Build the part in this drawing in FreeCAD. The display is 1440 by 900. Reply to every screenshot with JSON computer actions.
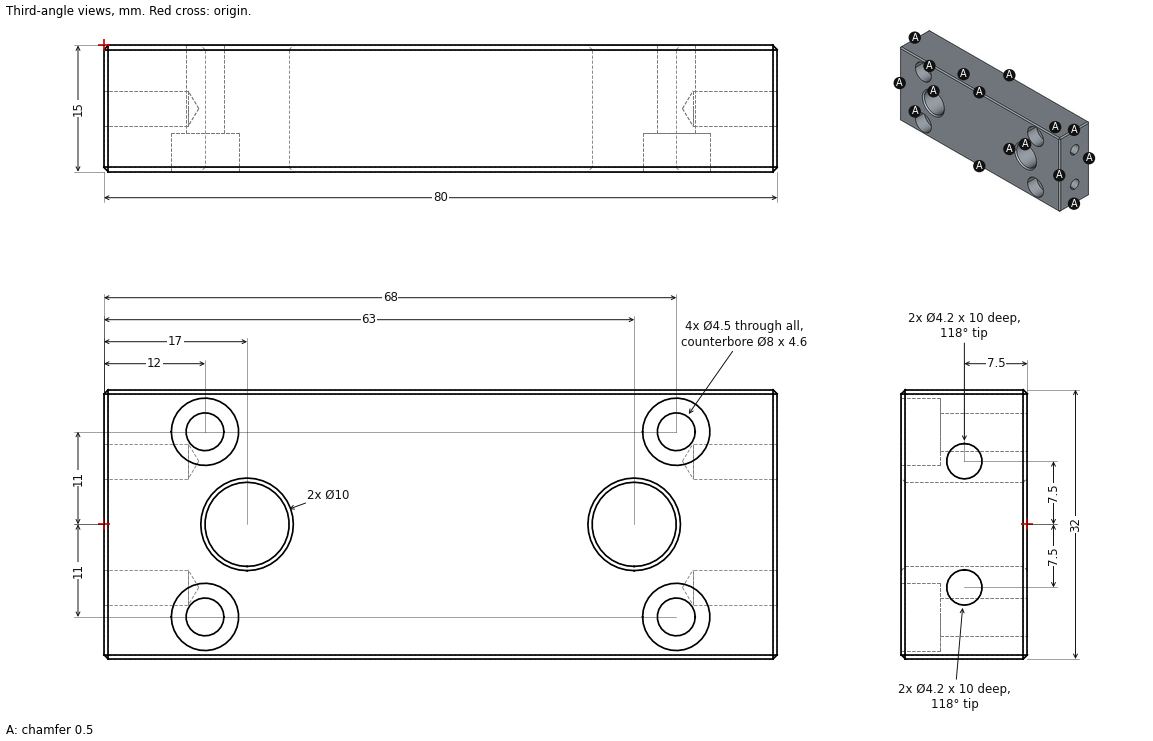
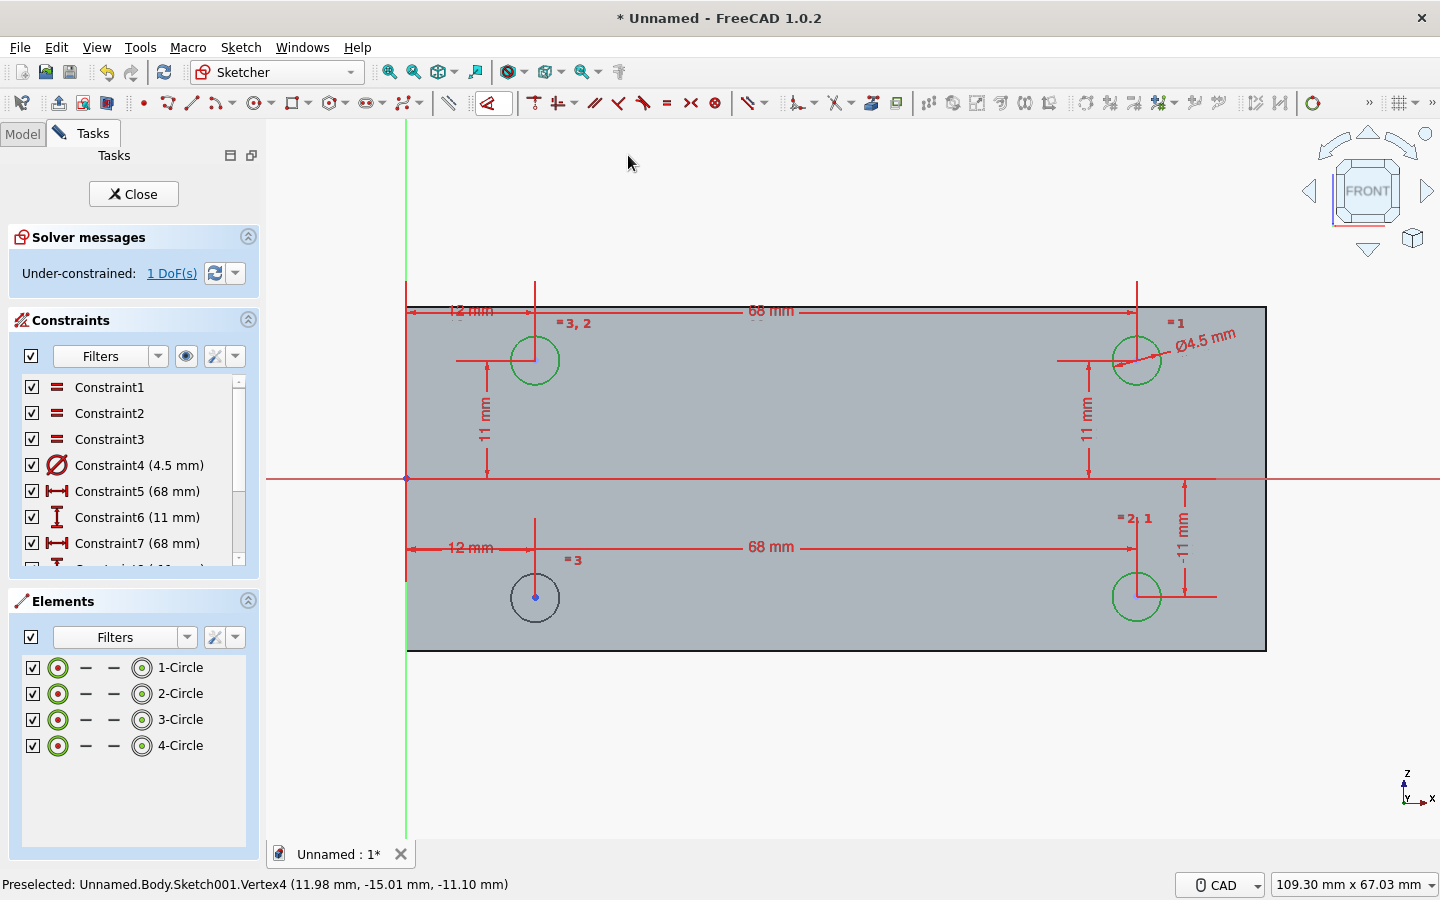
{"action": "left_click", "coordinate": [535, 598]}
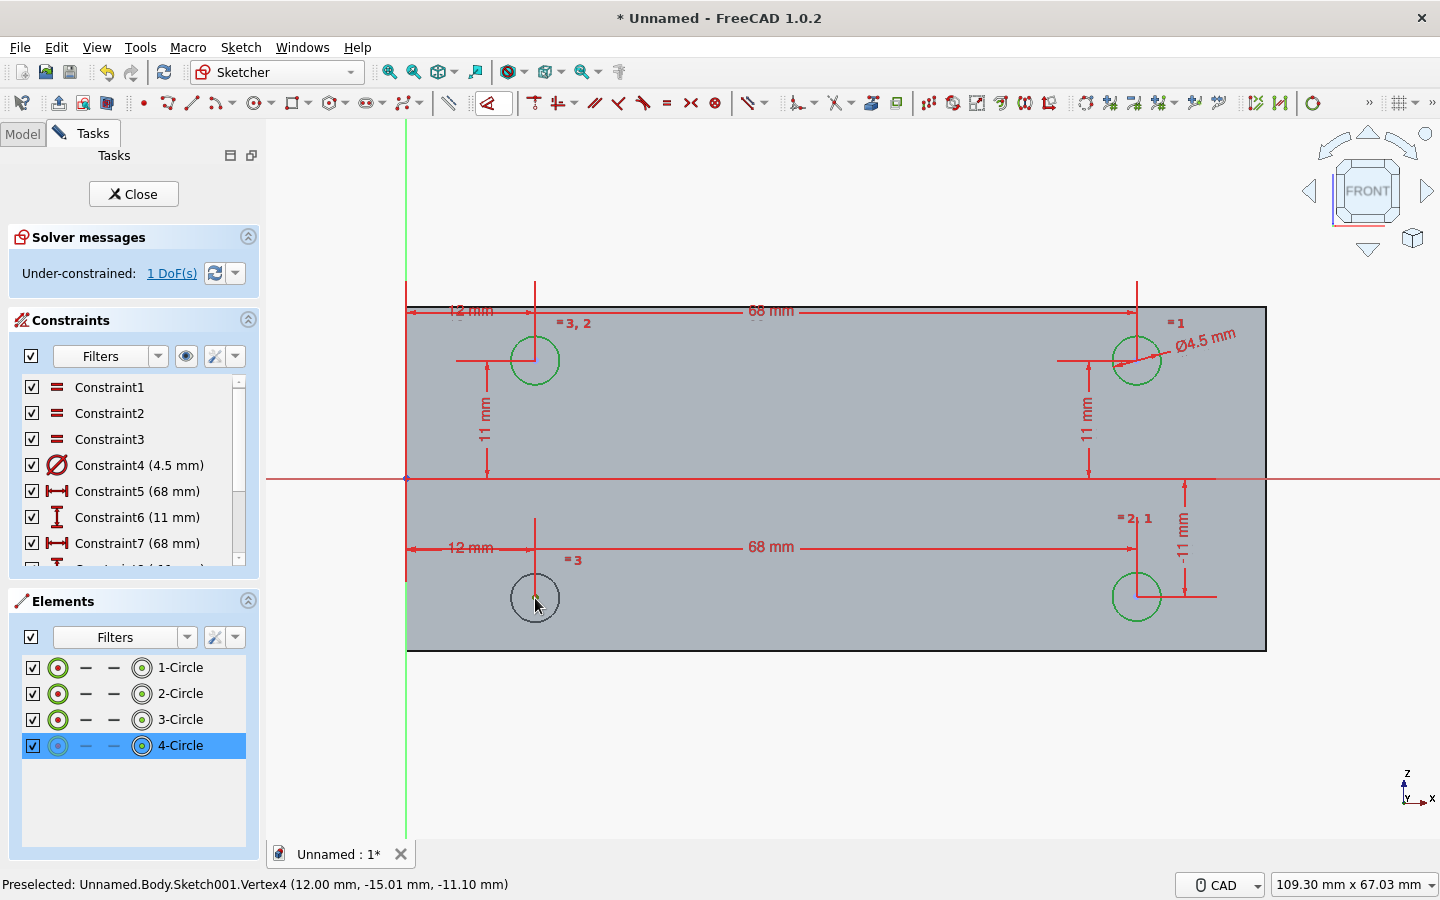
{"action": "key", "text": "i"}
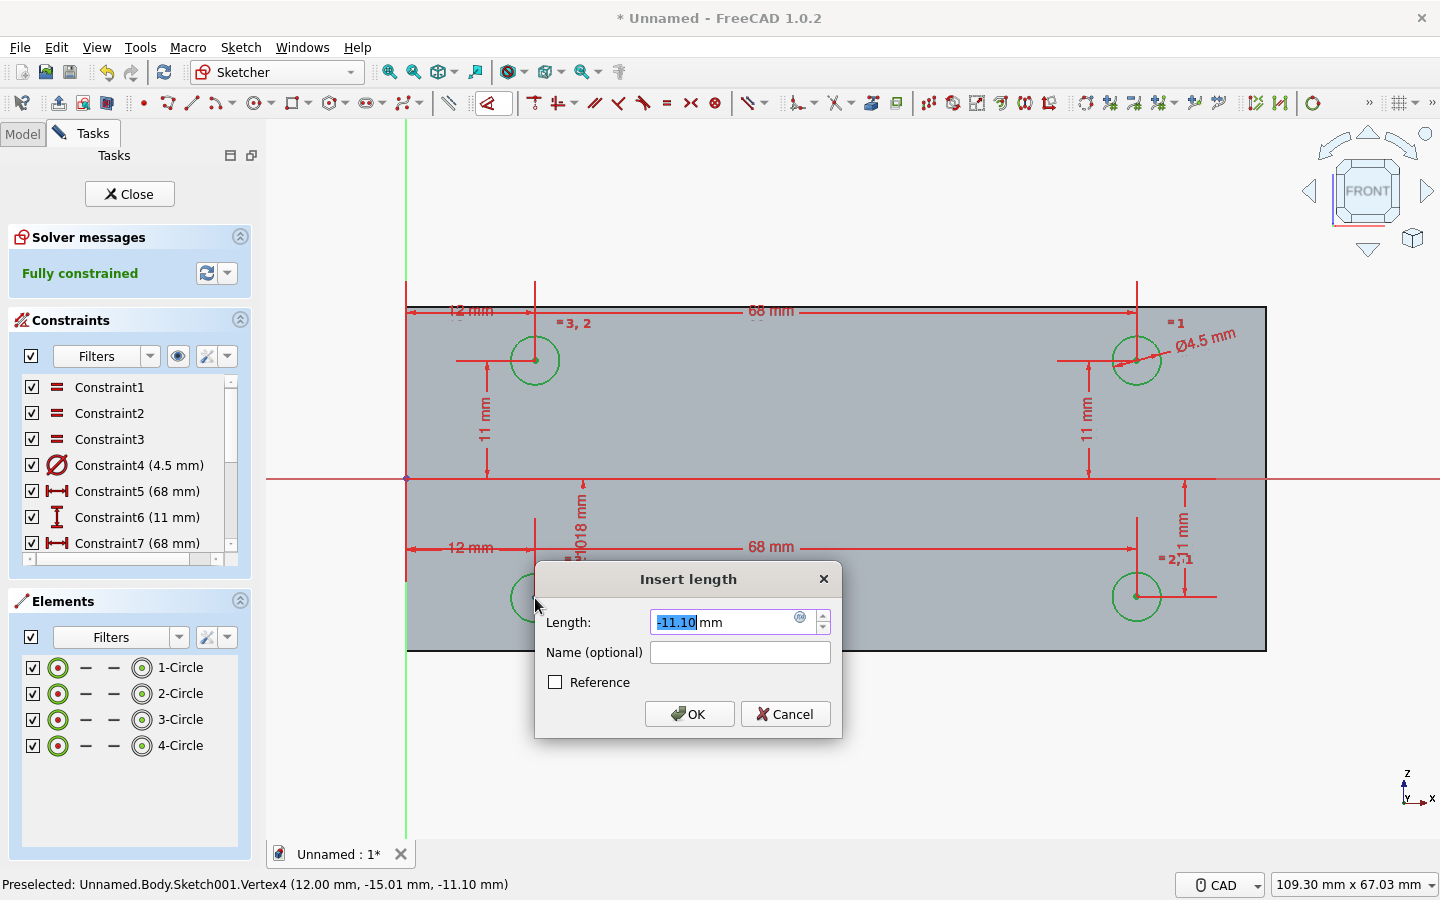
{"action": "type", "text": "-11"}
{"action": "key", "text": "Return"}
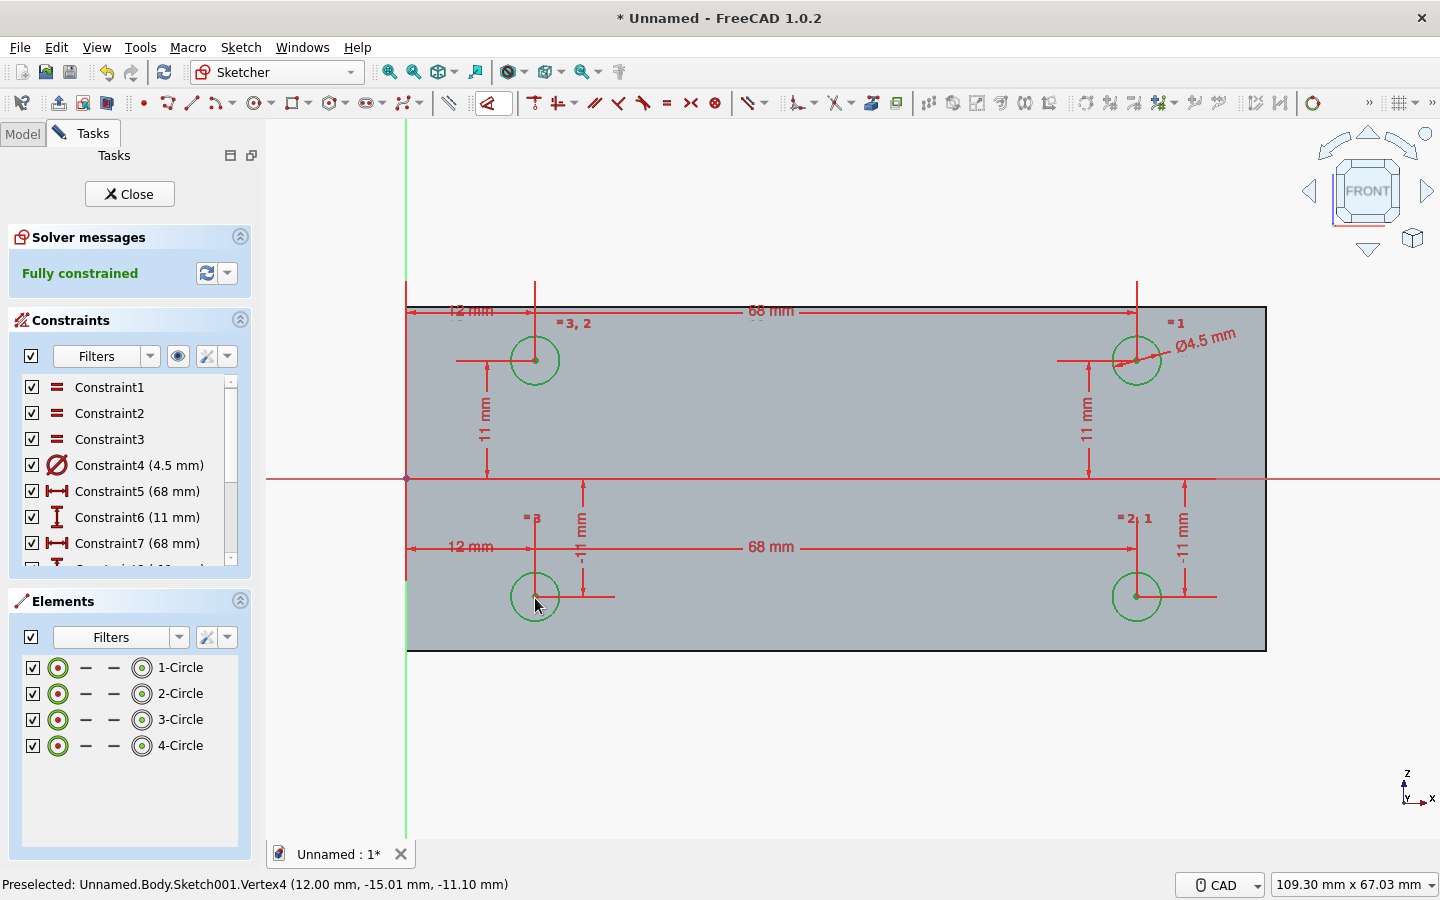
{"action": "left_click", "coordinate": [130, 194]}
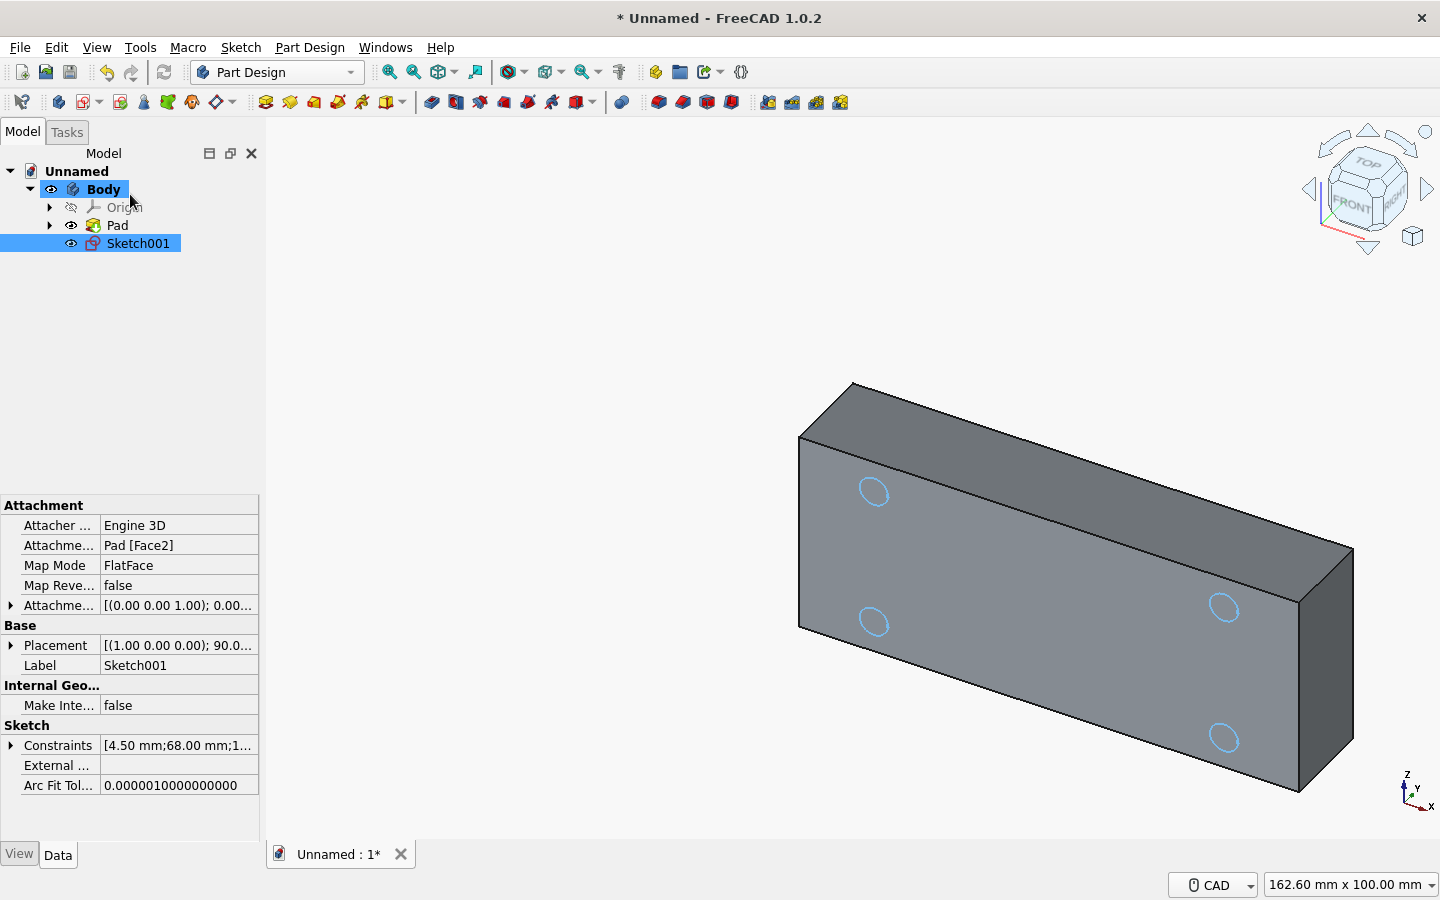
{"action": "left_click", "coordinate": [456, 102]}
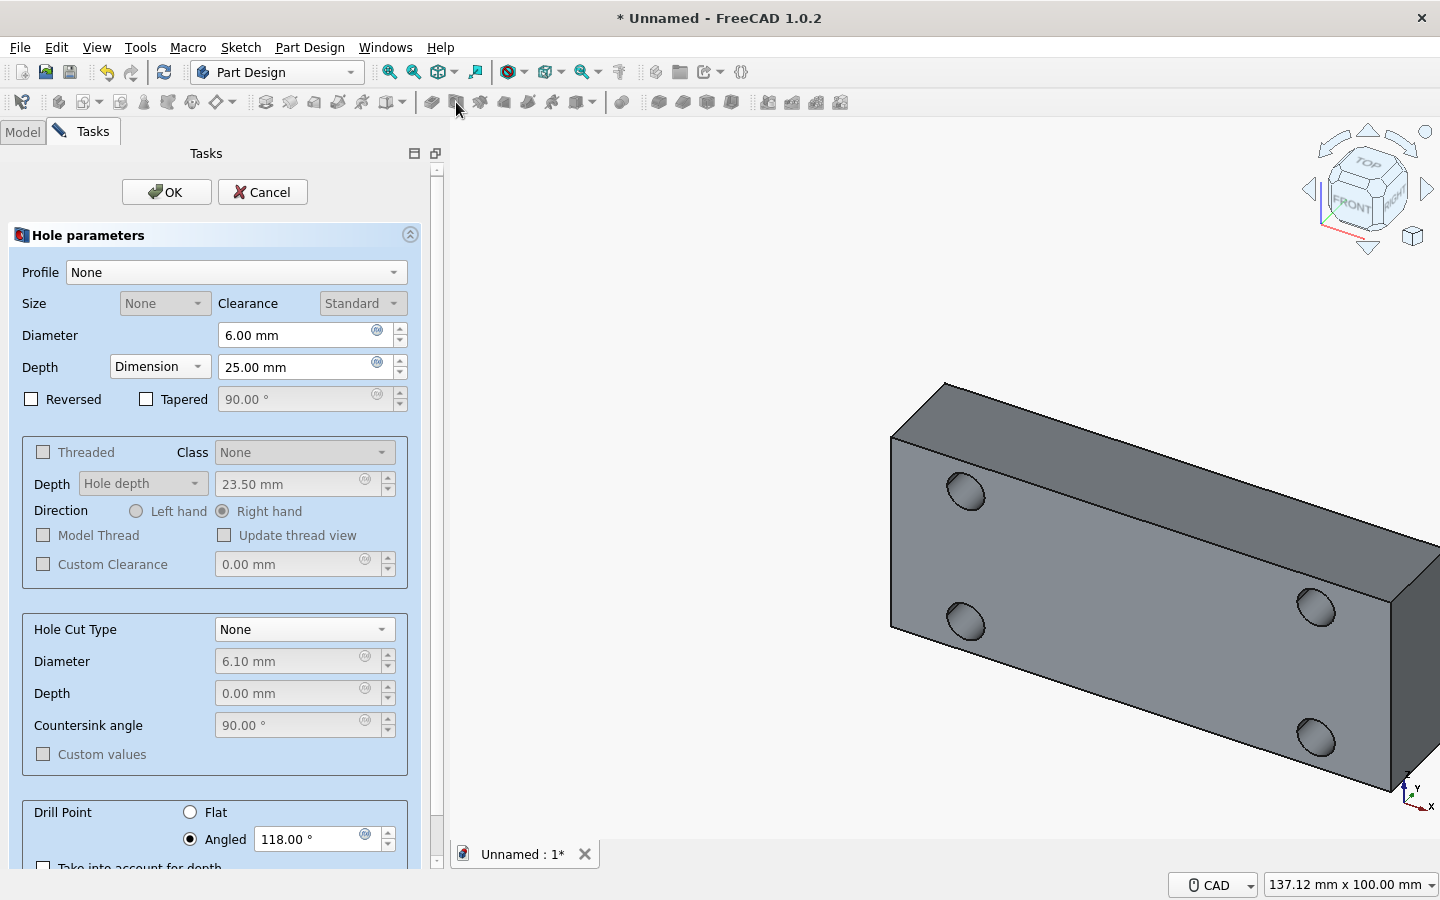
{"action": "triple_click", "coordinate": [305, 335]}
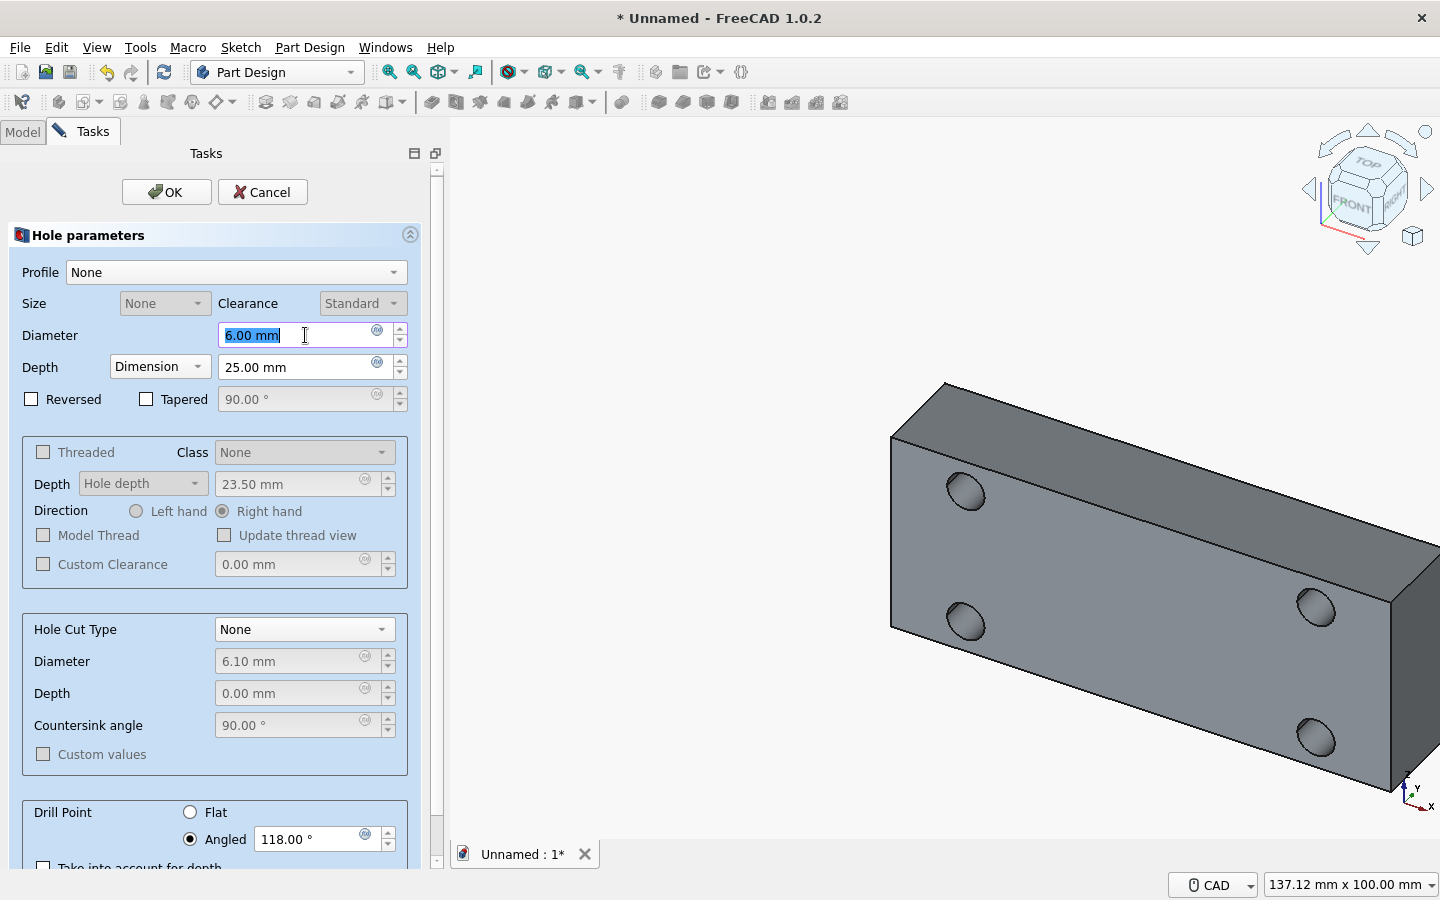
{"action": "type", "text": "4.5"}
{"action": "key", "text": "Tab"}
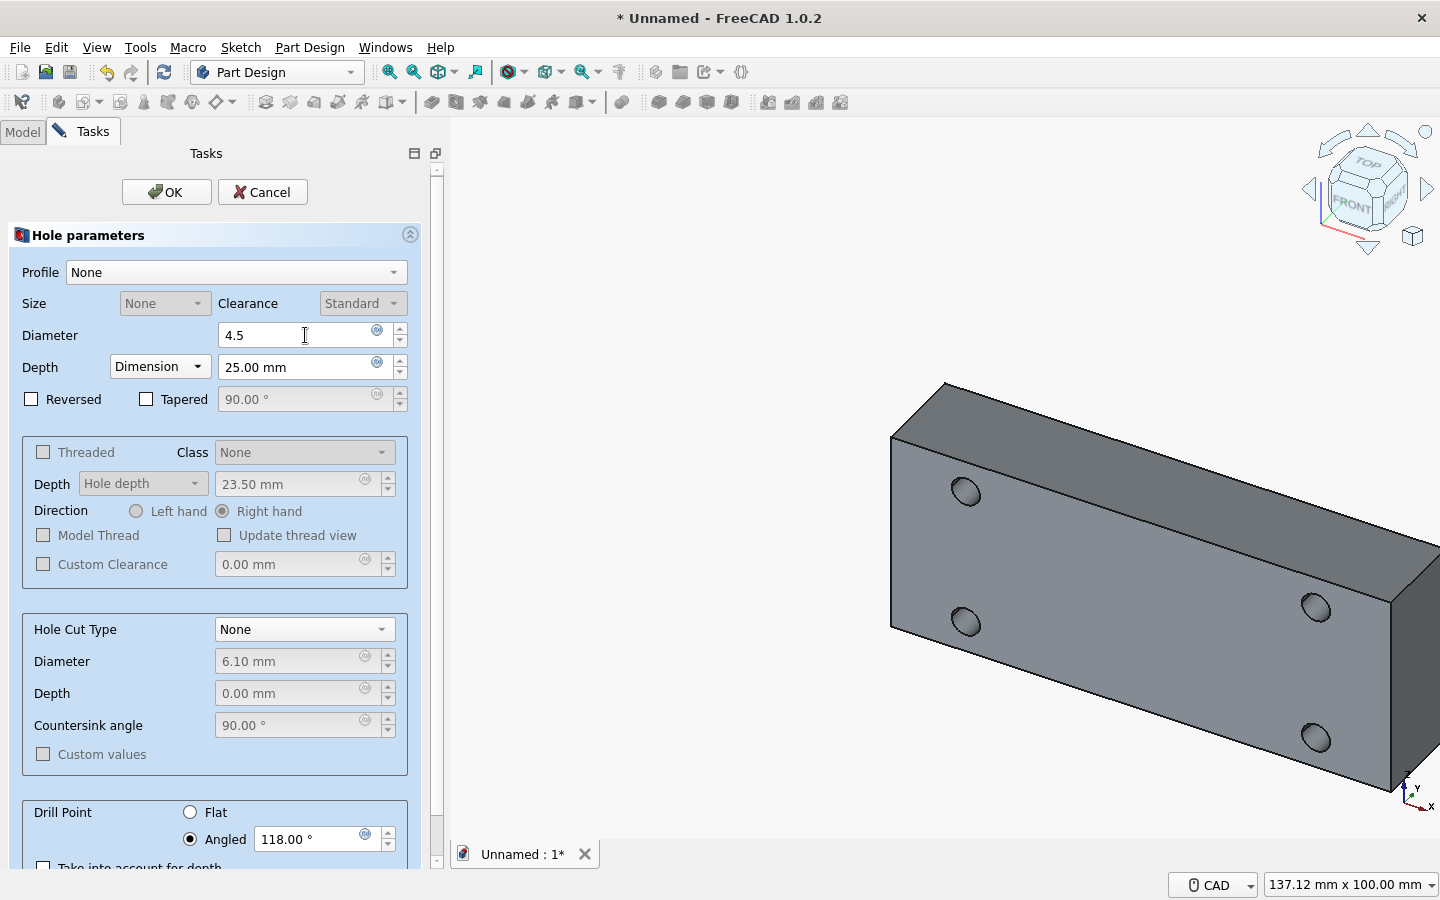
{"action": "left_click", "coordinate": [161, 366]}